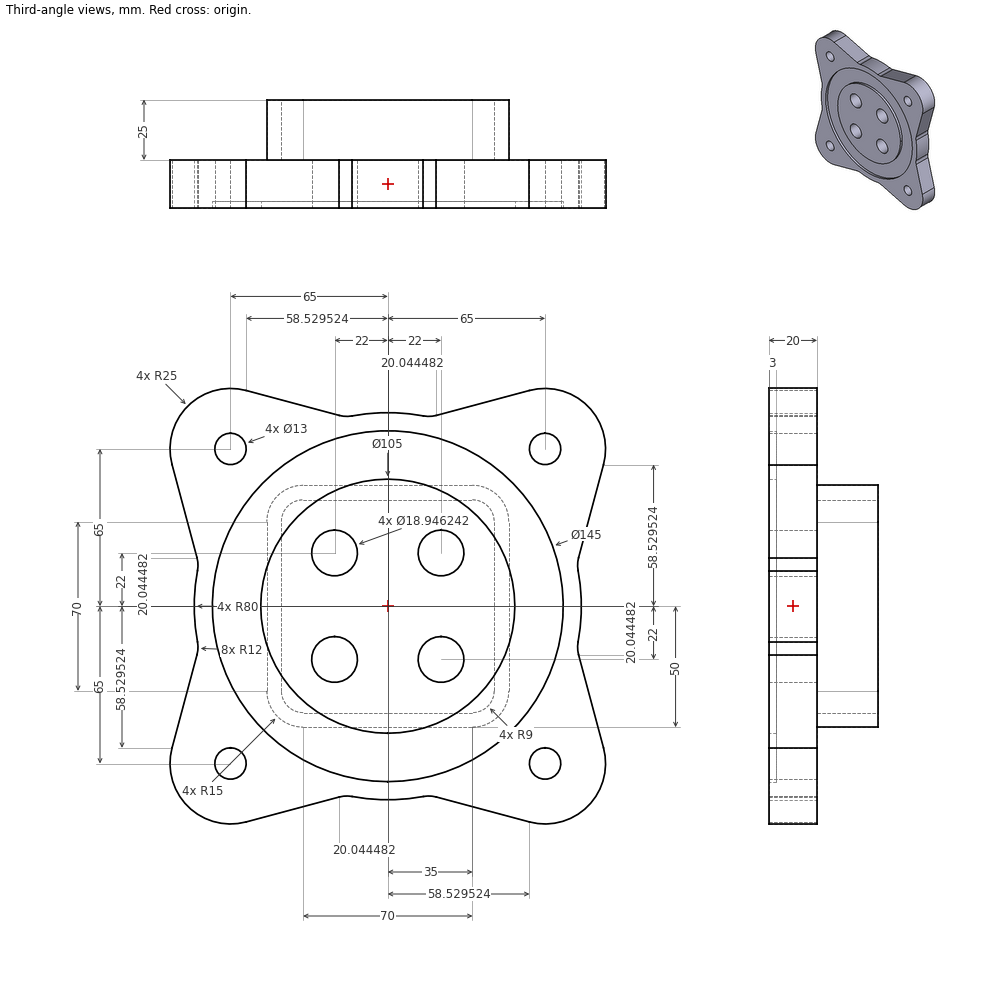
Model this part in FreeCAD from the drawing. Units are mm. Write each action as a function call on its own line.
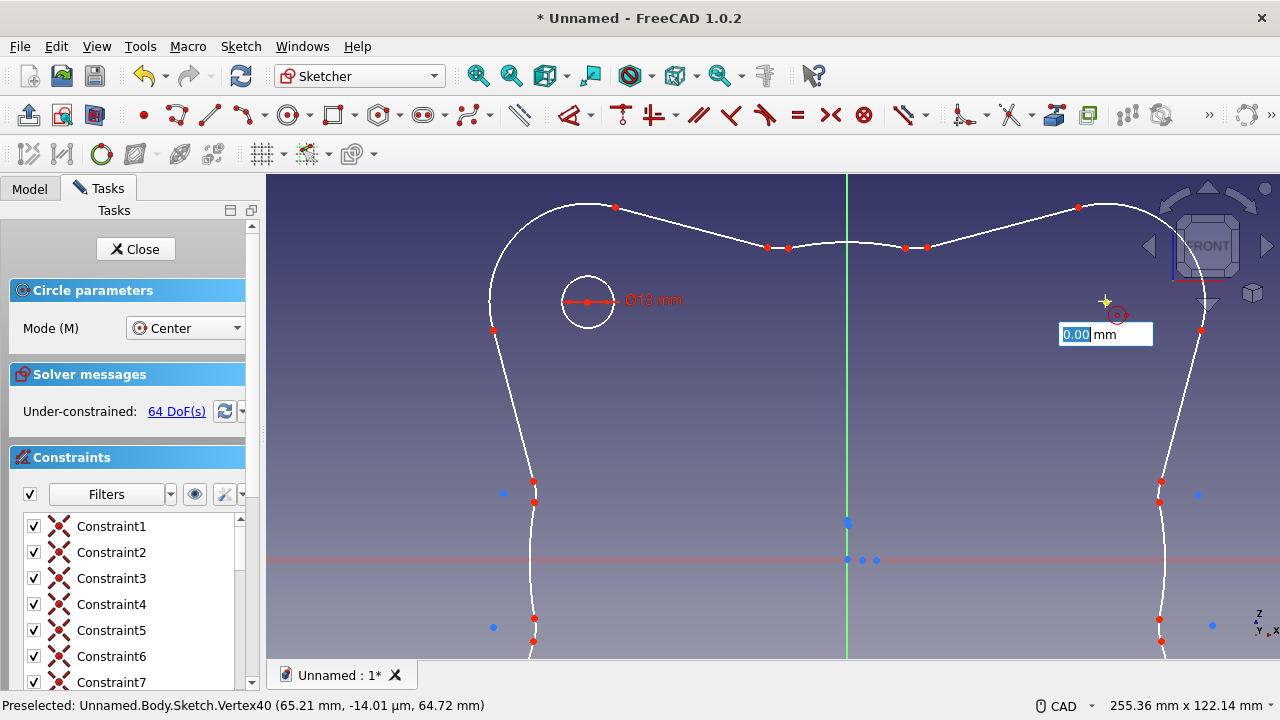
scroll(588, 300, down, 4)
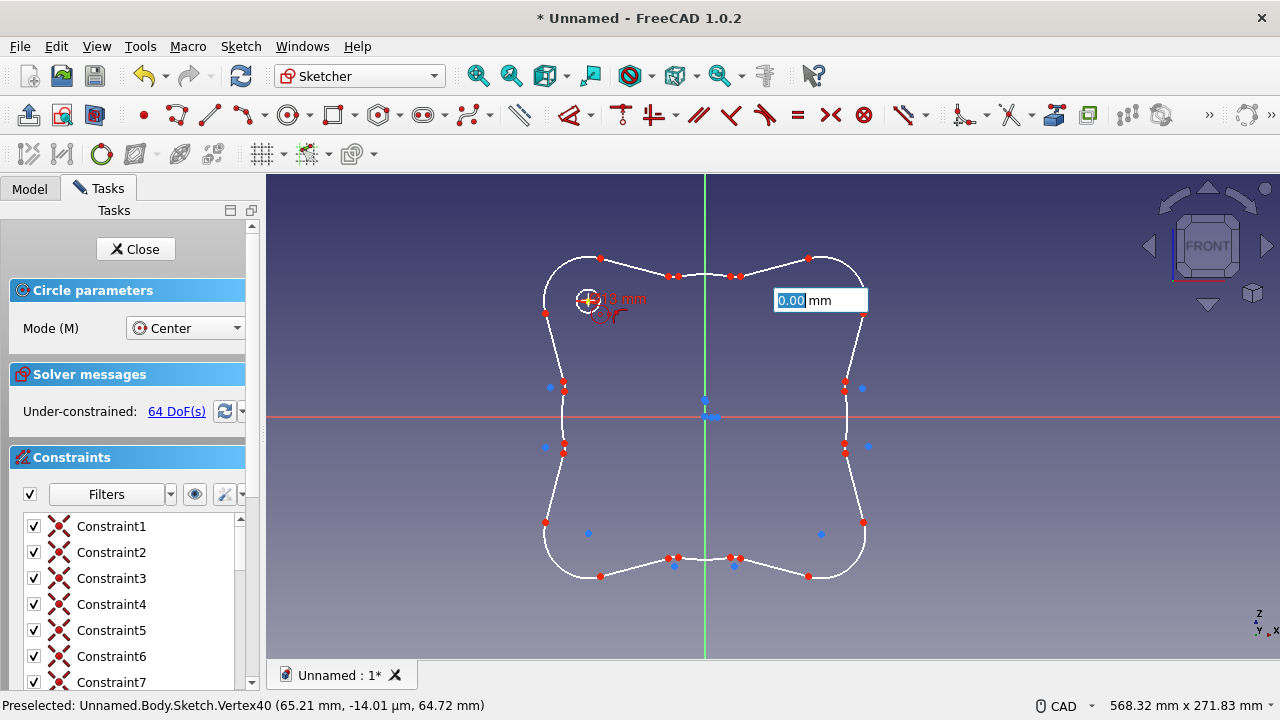
scroll(829, 293, up, 2)
move(829, 292)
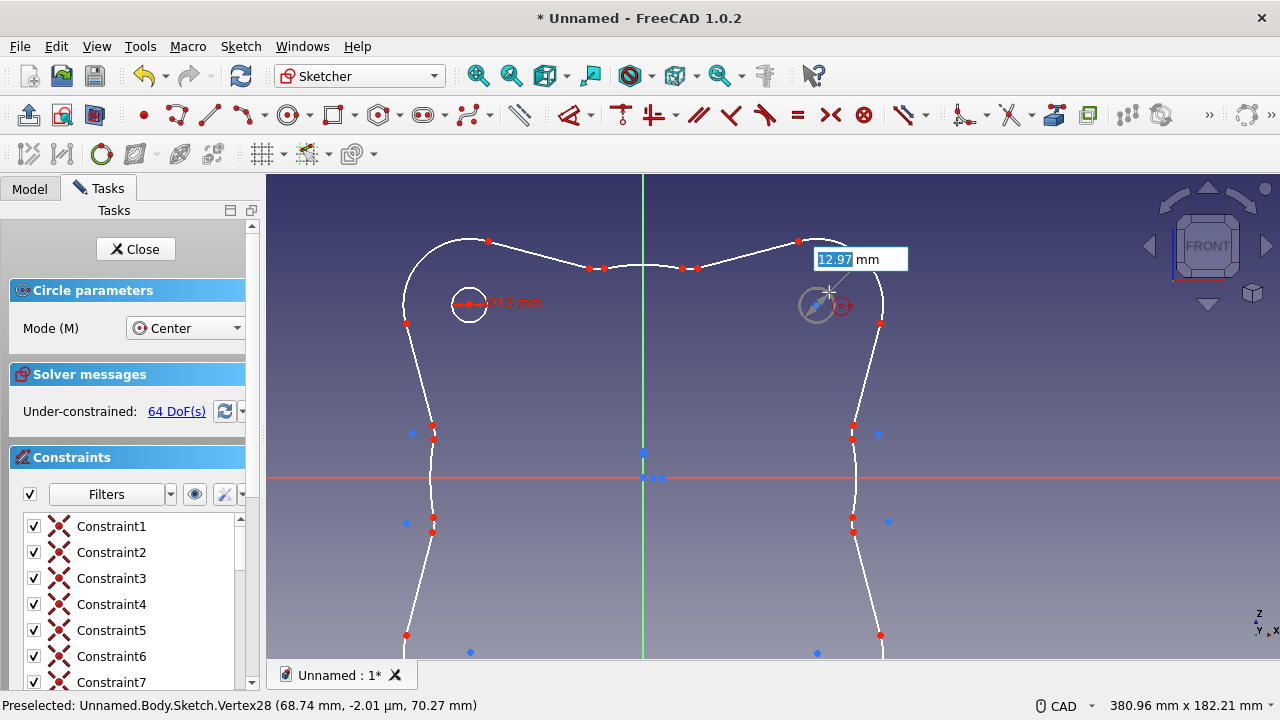
text(13)
key(Return)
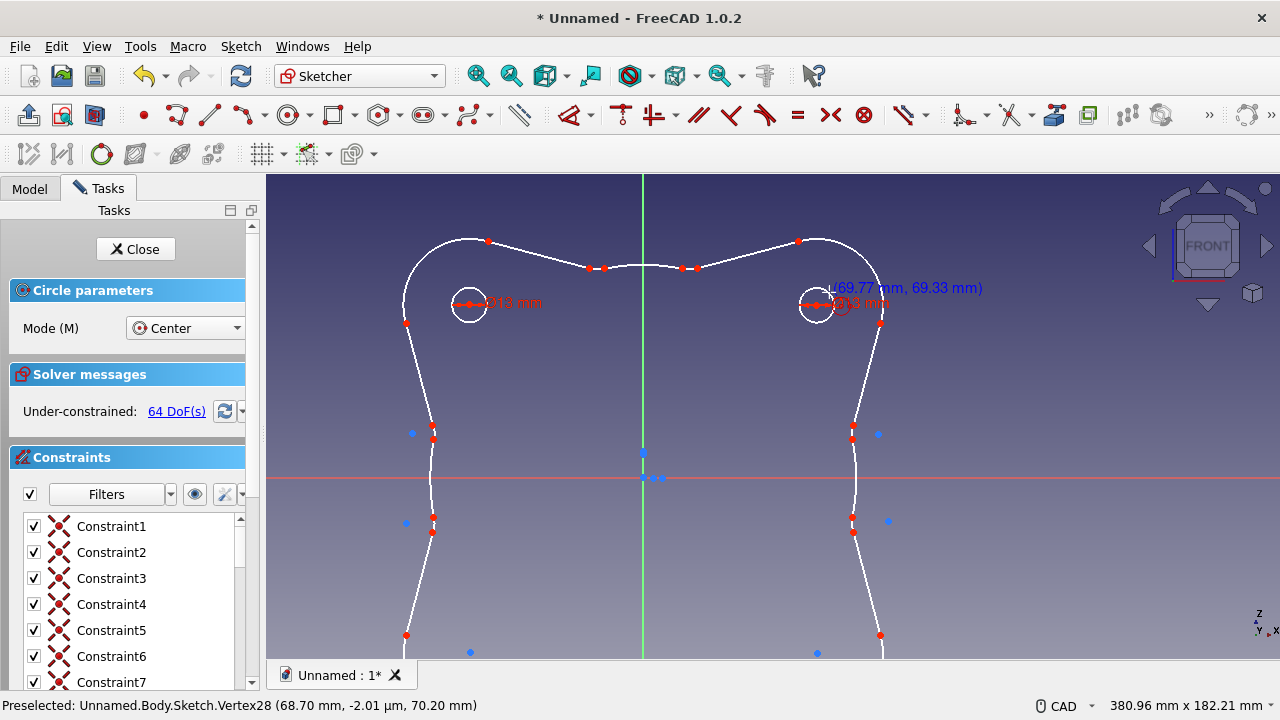
scroll(829, 292, down, 2)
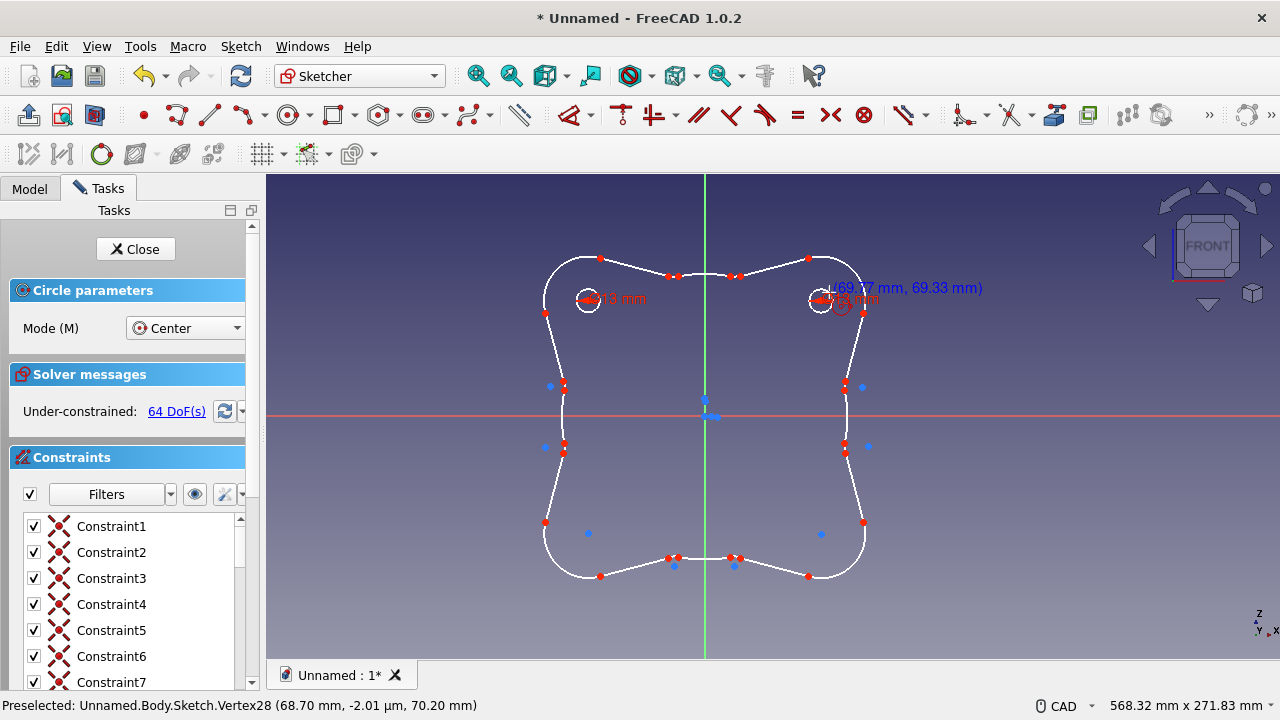
scroll(589, 532, up, 4)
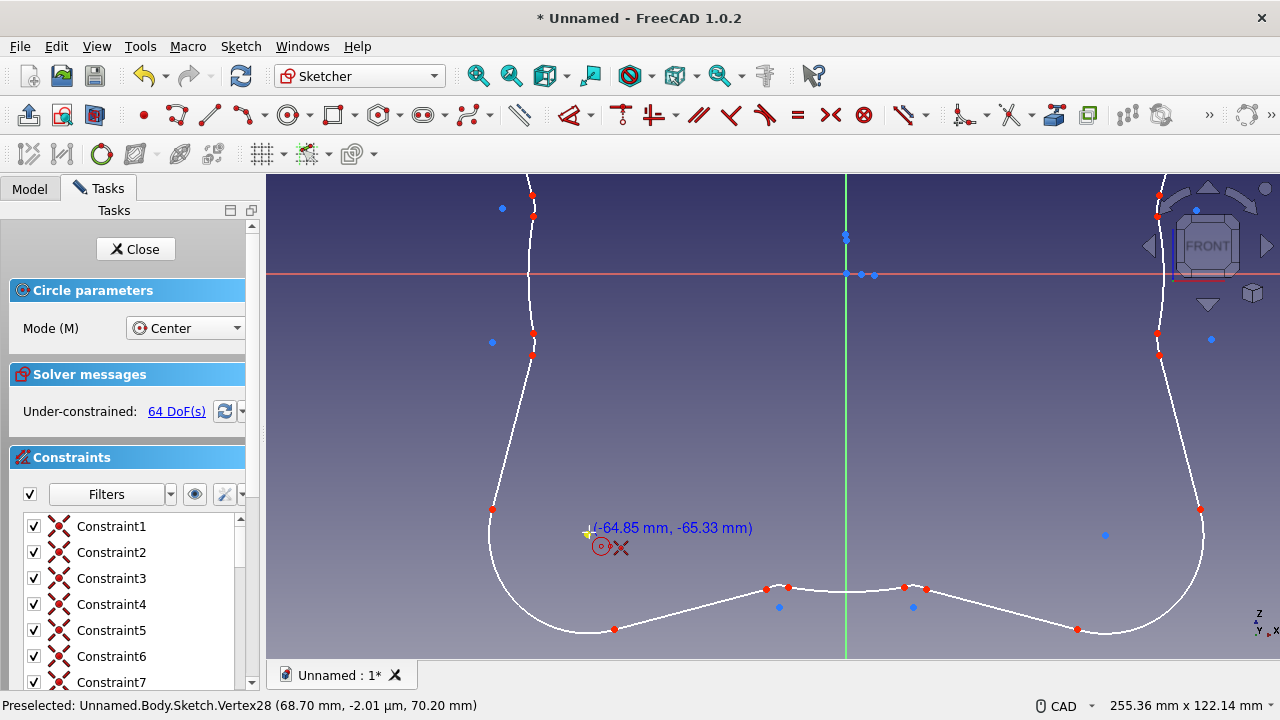
click(588, 532)
move(606, 514)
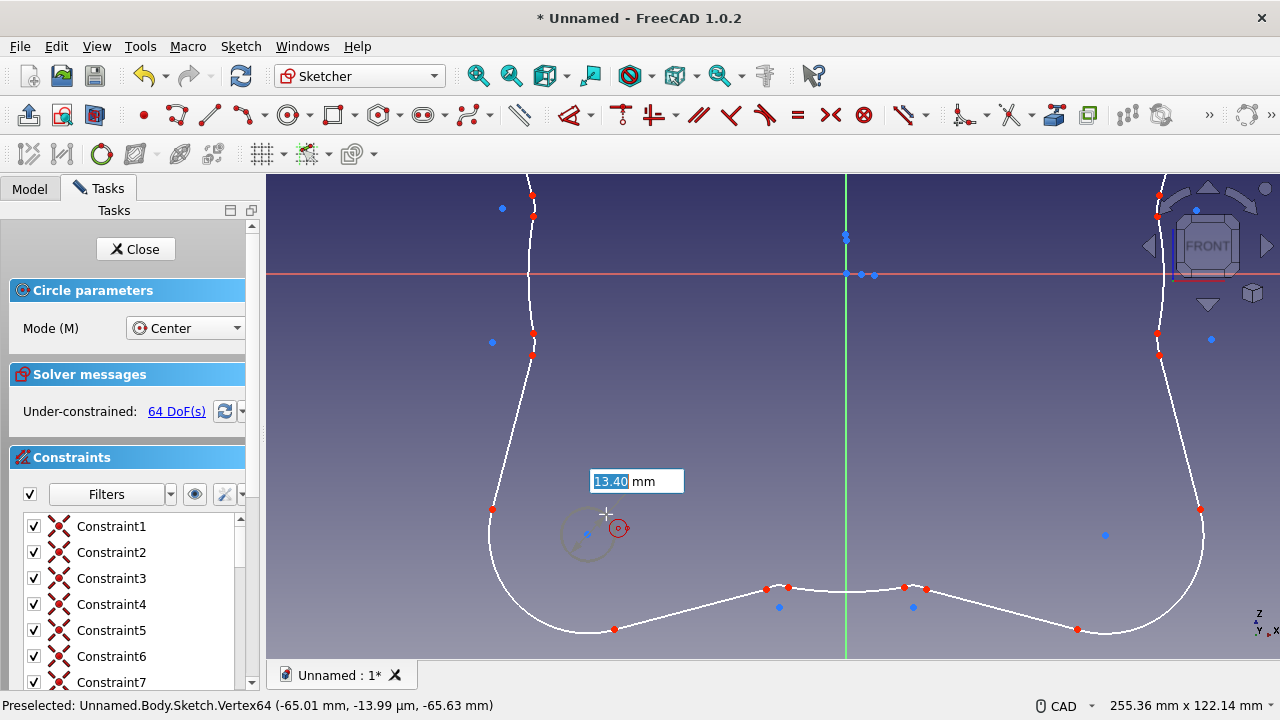
text(13)
key(Return)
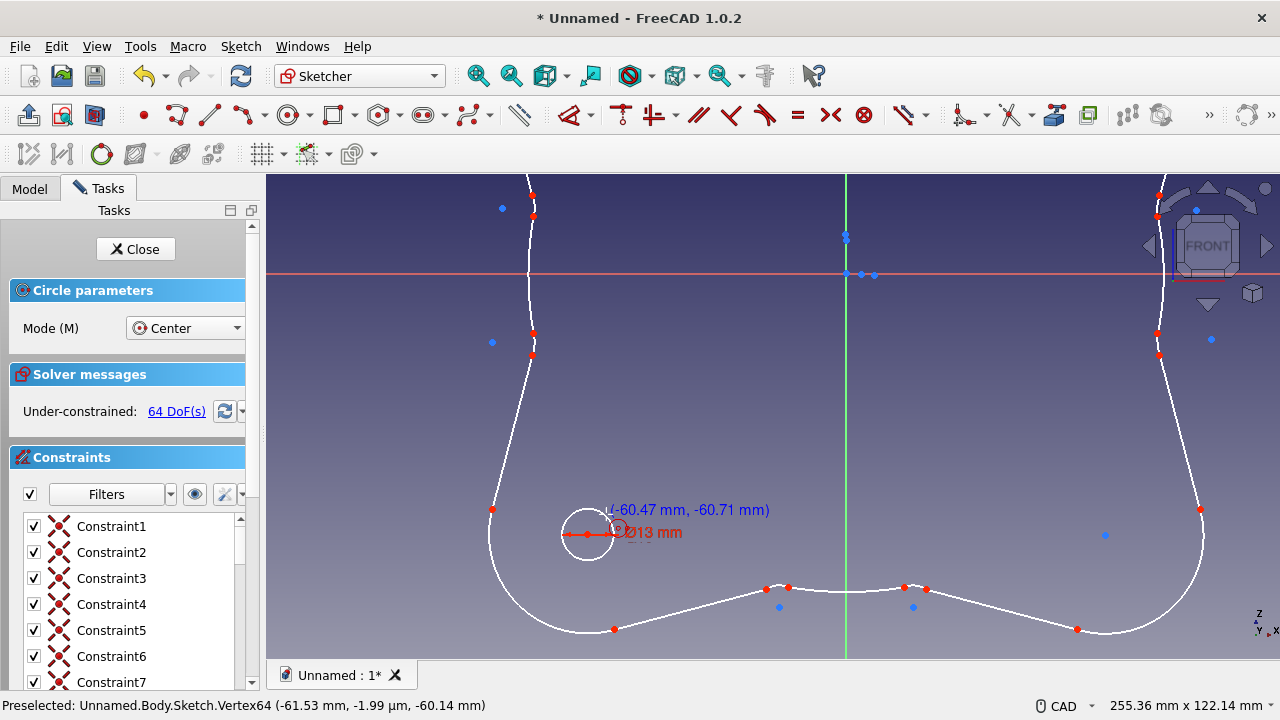
click(1104, 532)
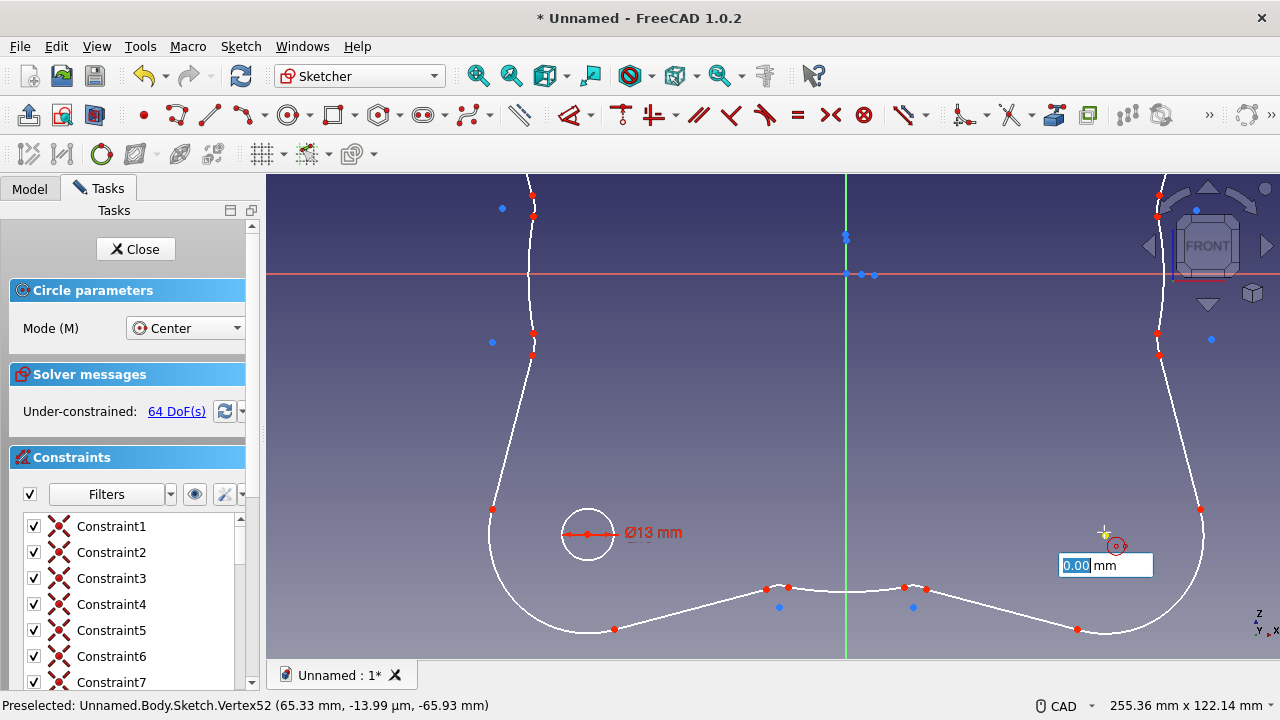
scroll(589, 533, down, 4)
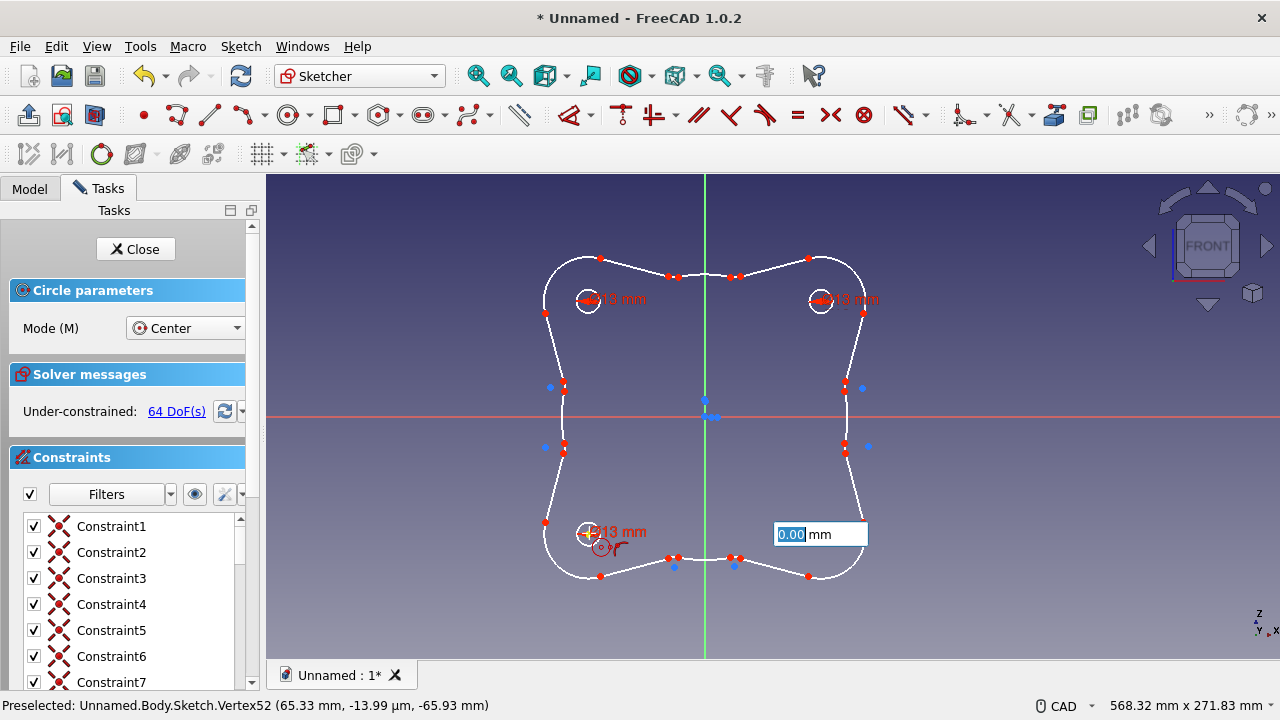
scroll(829, 525, up, 2)
move(829, 524)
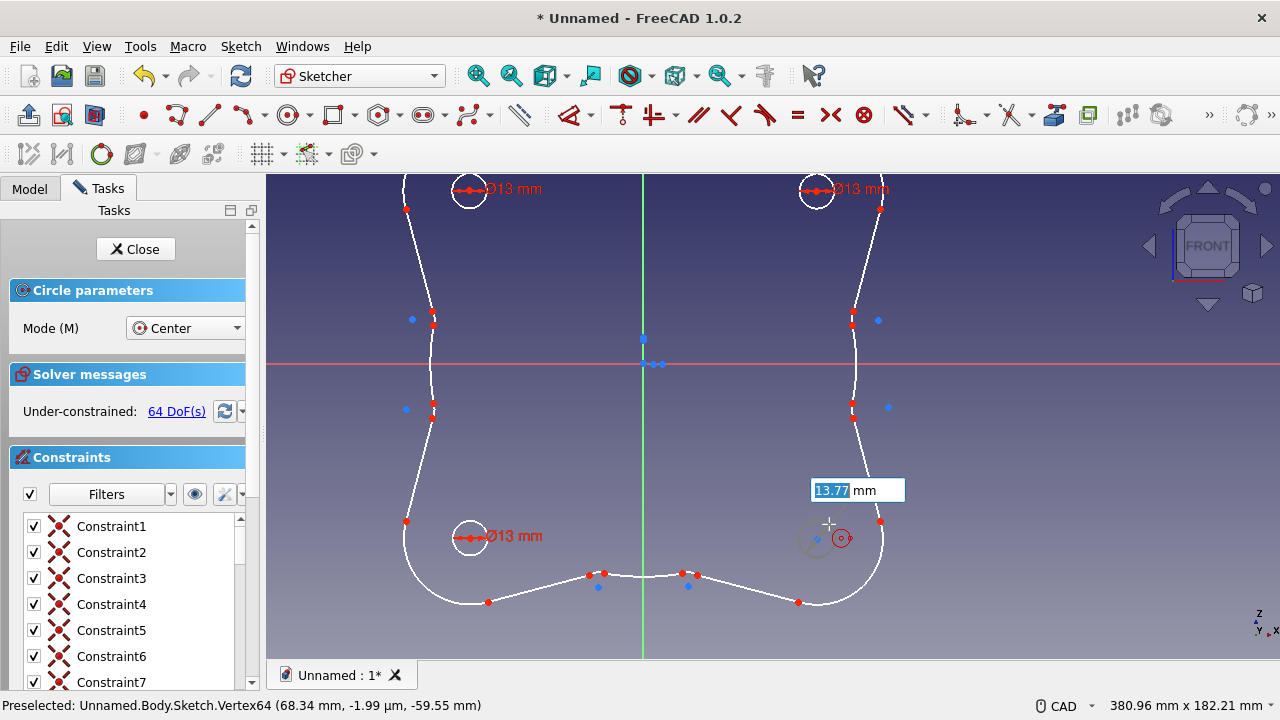
text(13)
key(Return)
key(Escape)